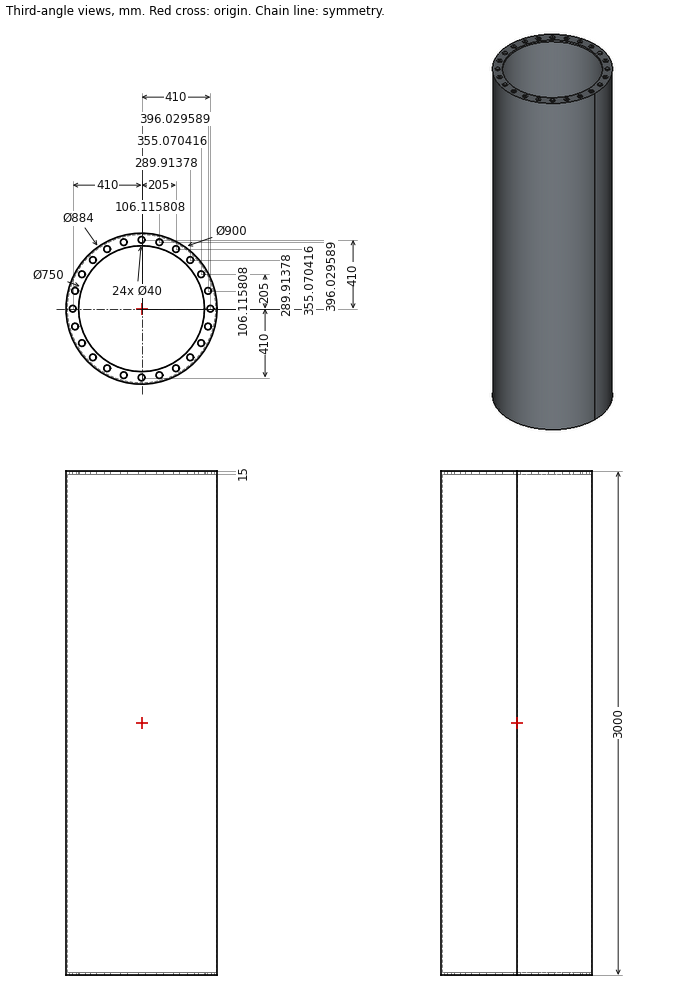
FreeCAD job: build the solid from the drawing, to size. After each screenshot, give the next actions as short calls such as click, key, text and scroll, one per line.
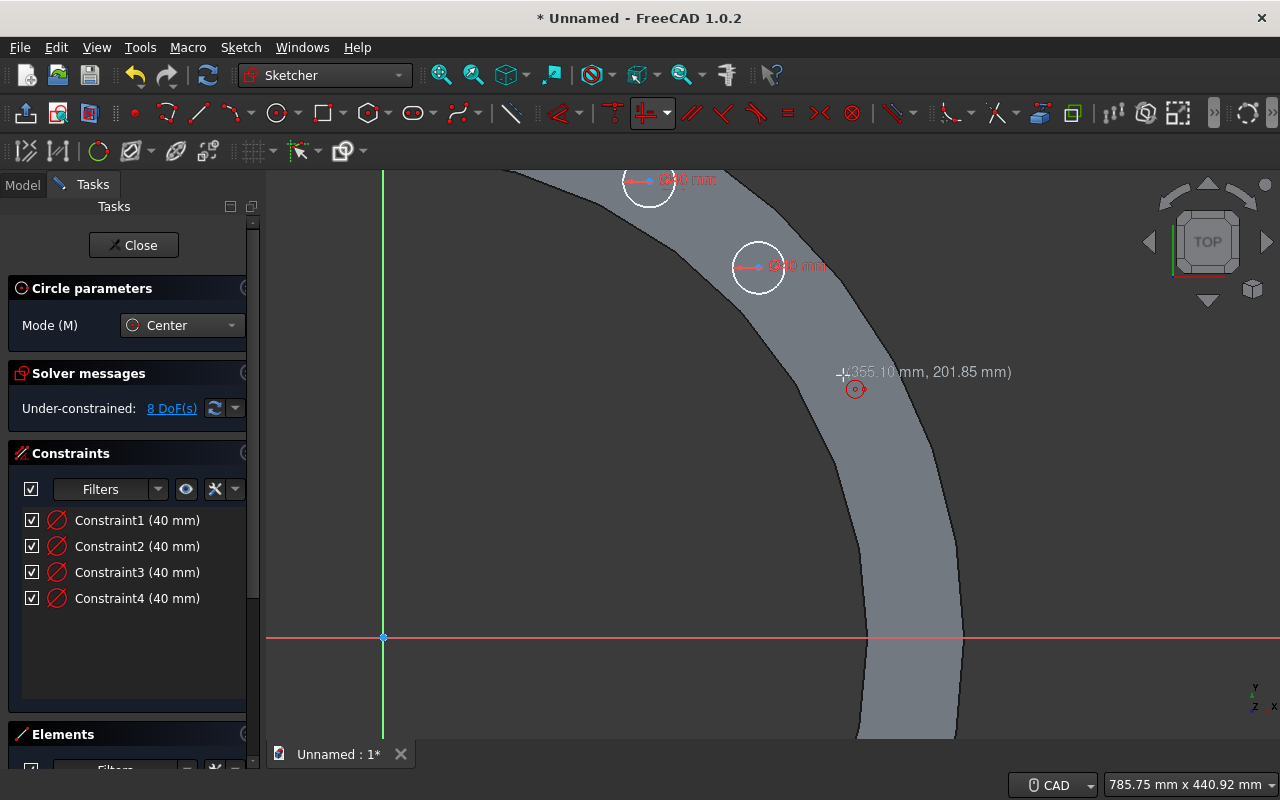
scroll(843, 375, down, 6)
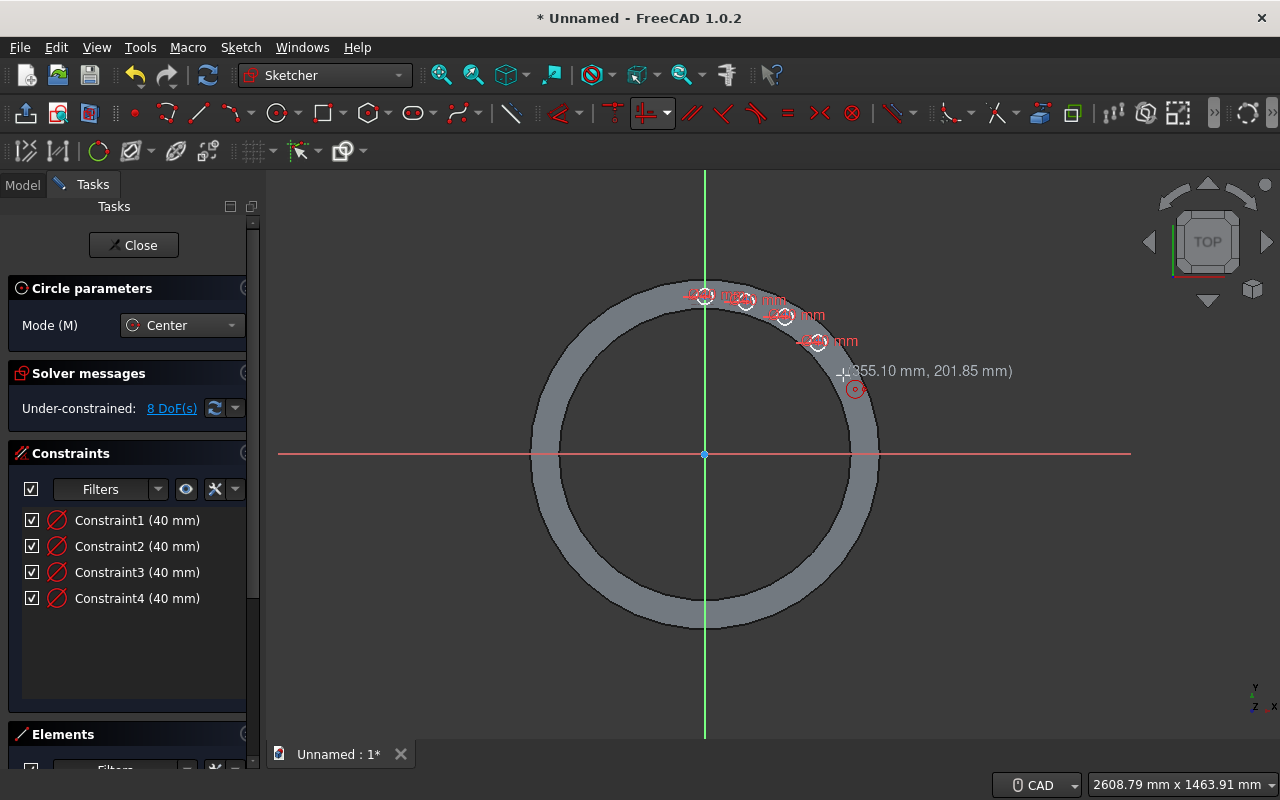
click(843, 375)
move(848, 369)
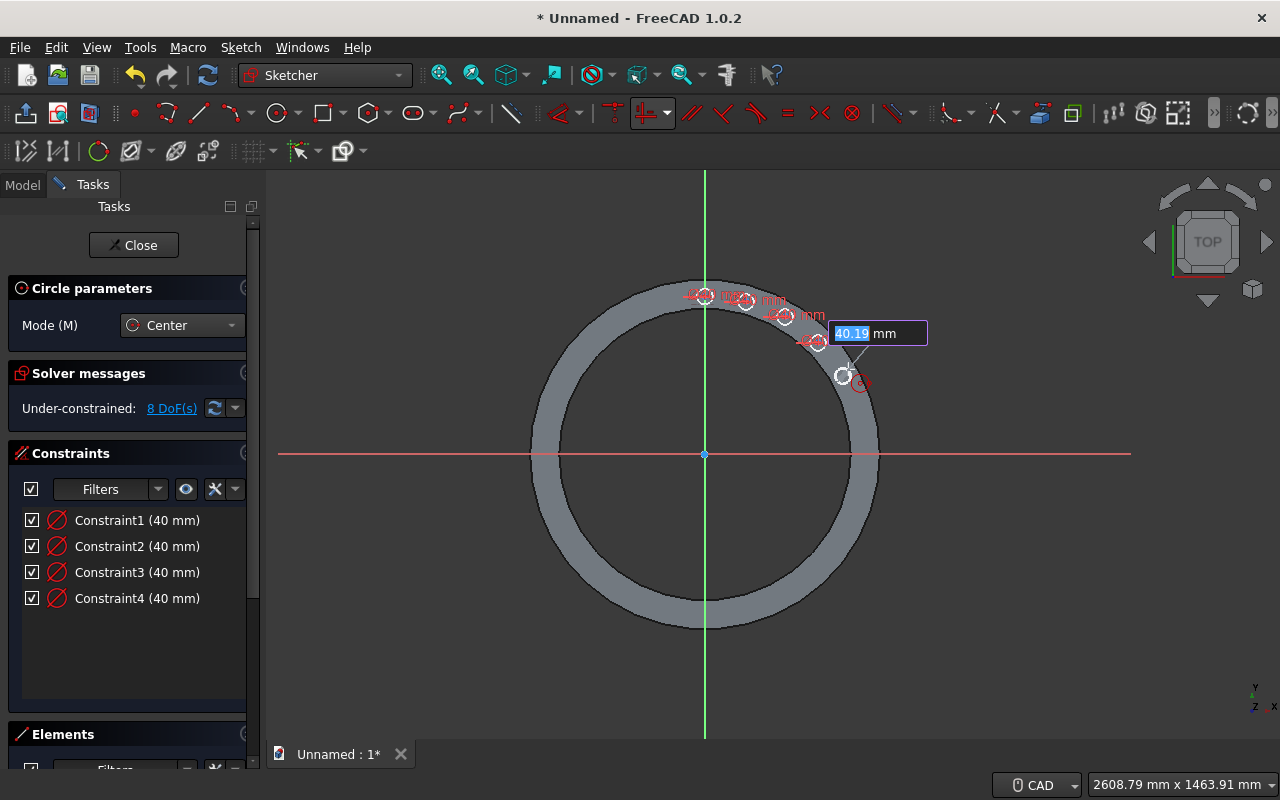
text(40)
key(Return)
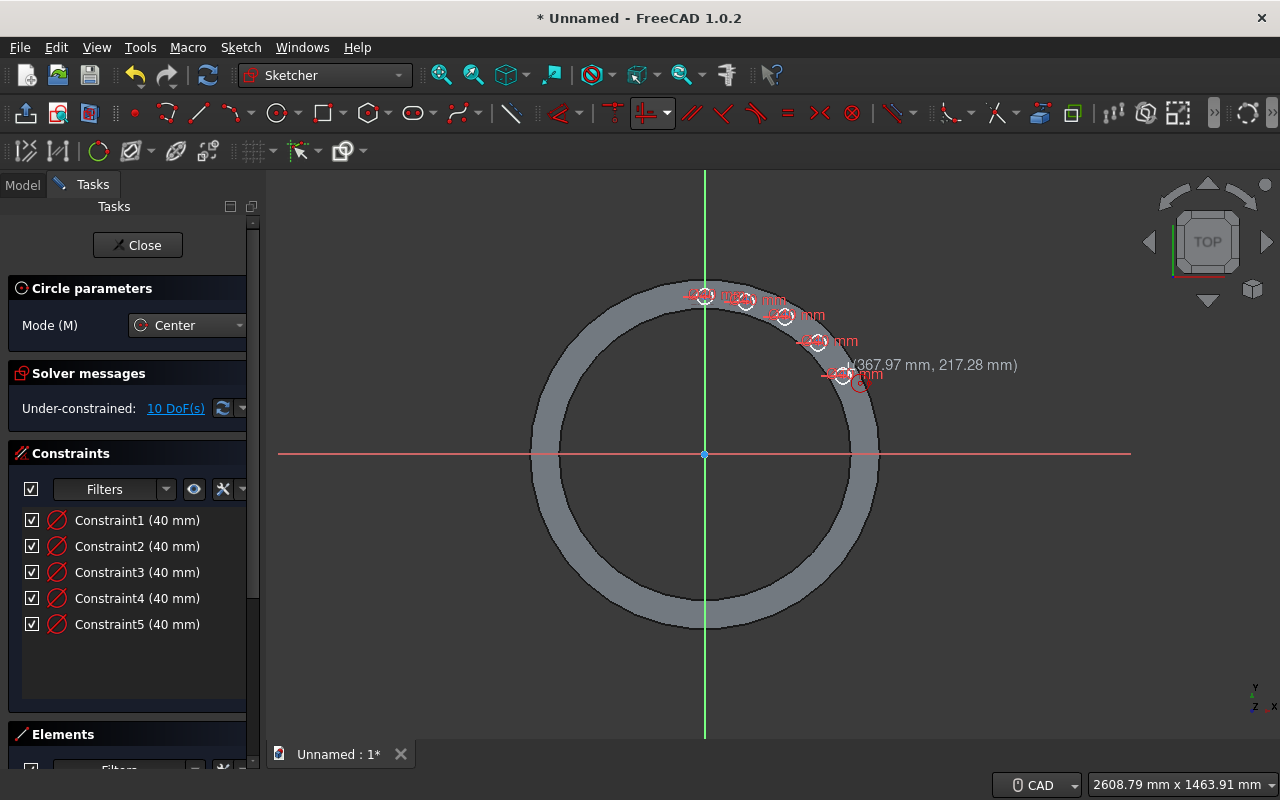
scroll(859, 413, up, 6)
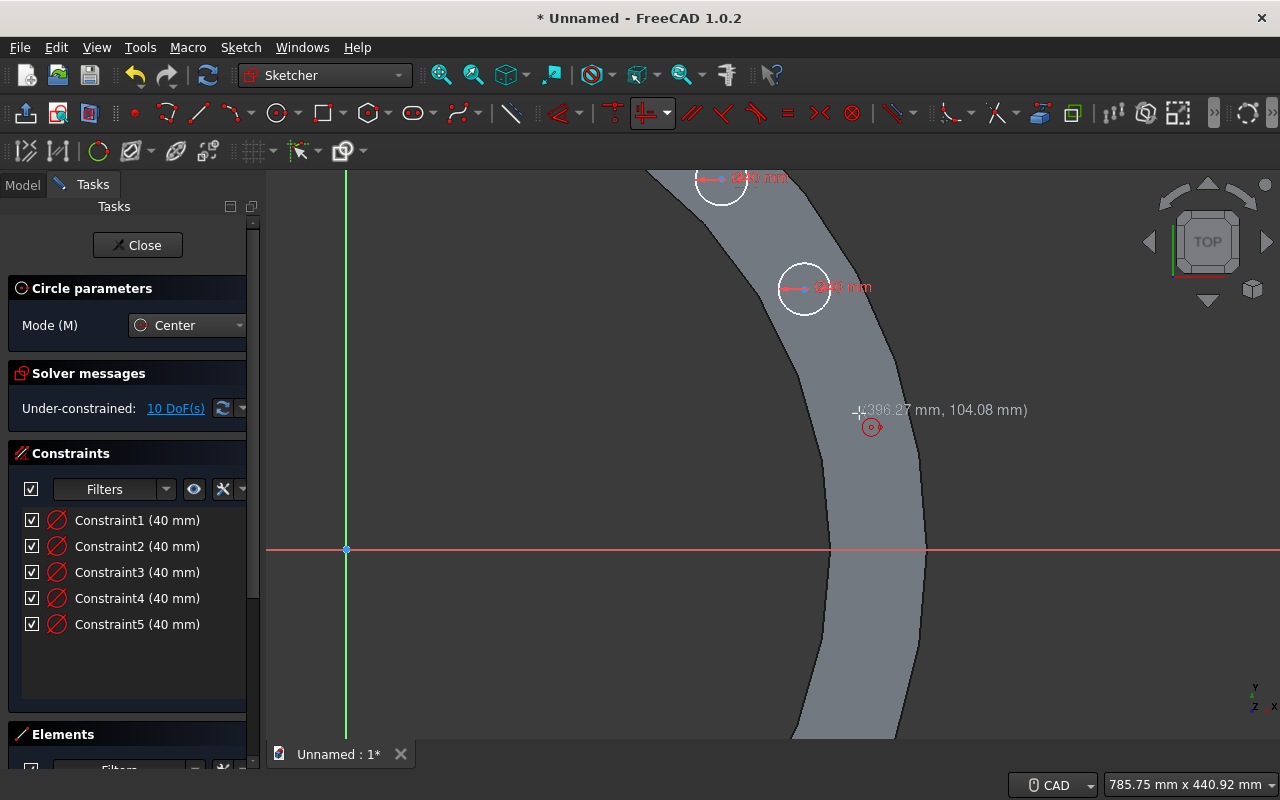
scroll(859, 413, down, 6)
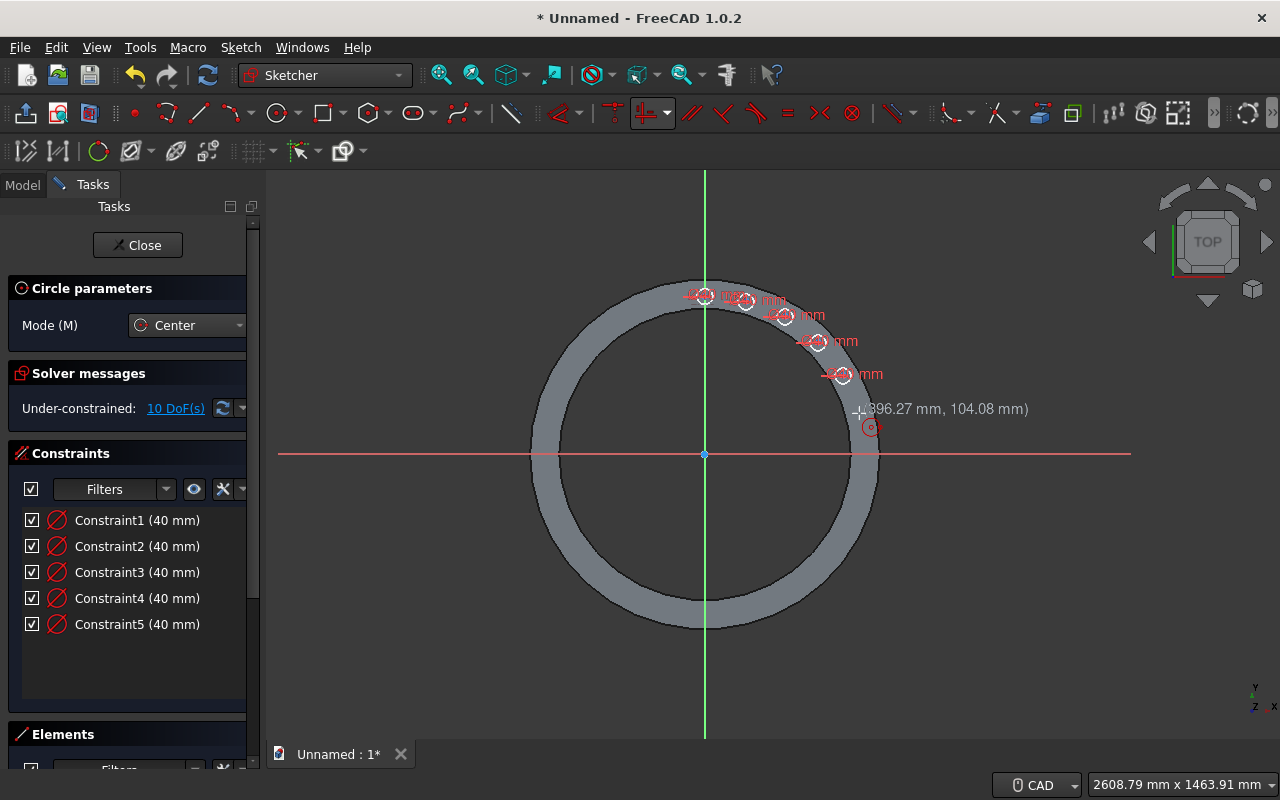
click(859, 413)
move(864, 408)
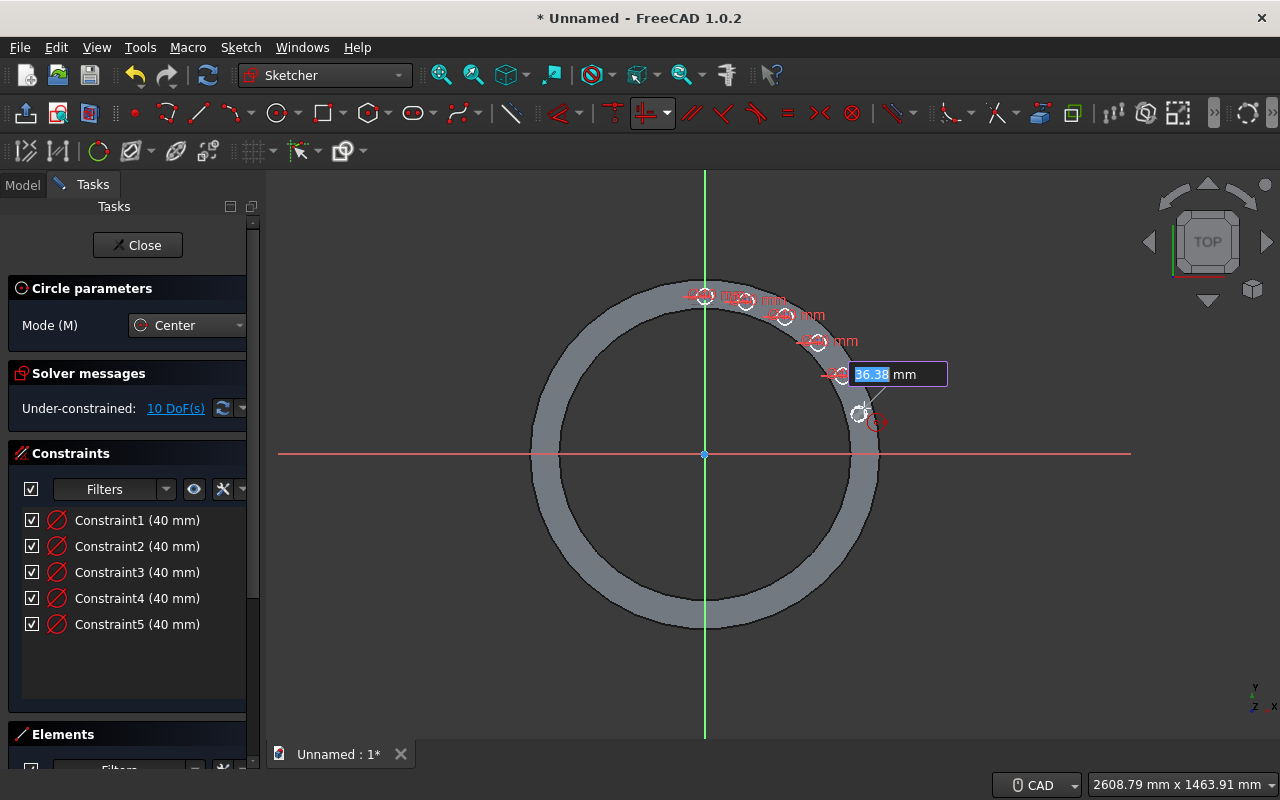
text(40)
key(Return)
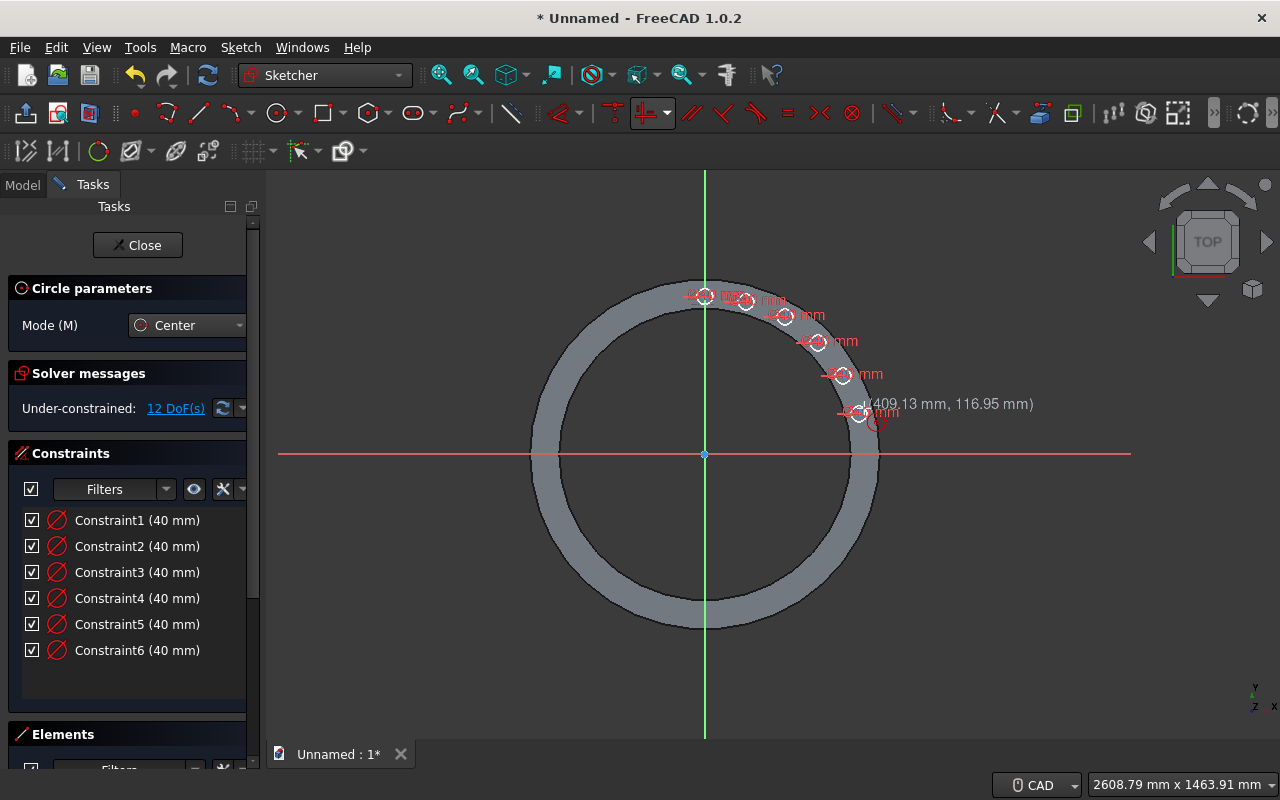
scroll(864, 454, up, 6)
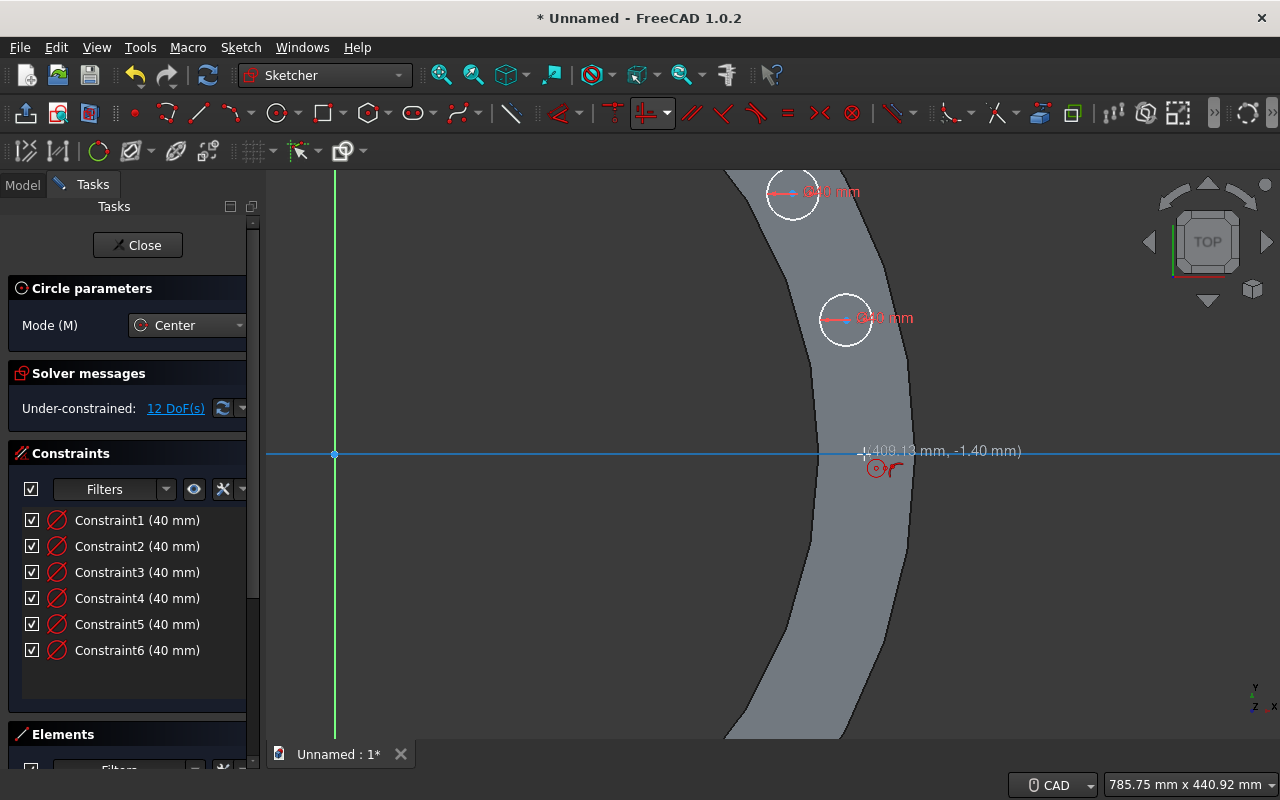
scroll(864, 455, down, 6)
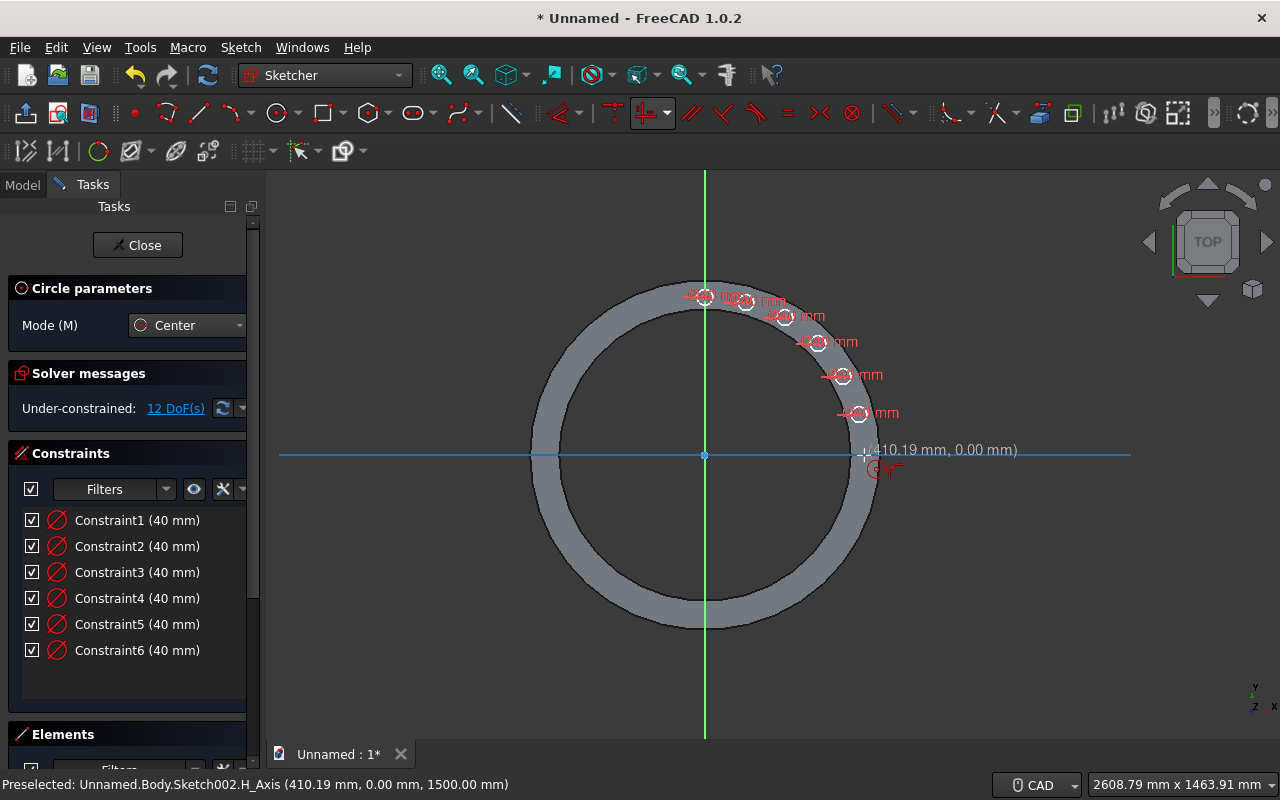
click(864, 455)